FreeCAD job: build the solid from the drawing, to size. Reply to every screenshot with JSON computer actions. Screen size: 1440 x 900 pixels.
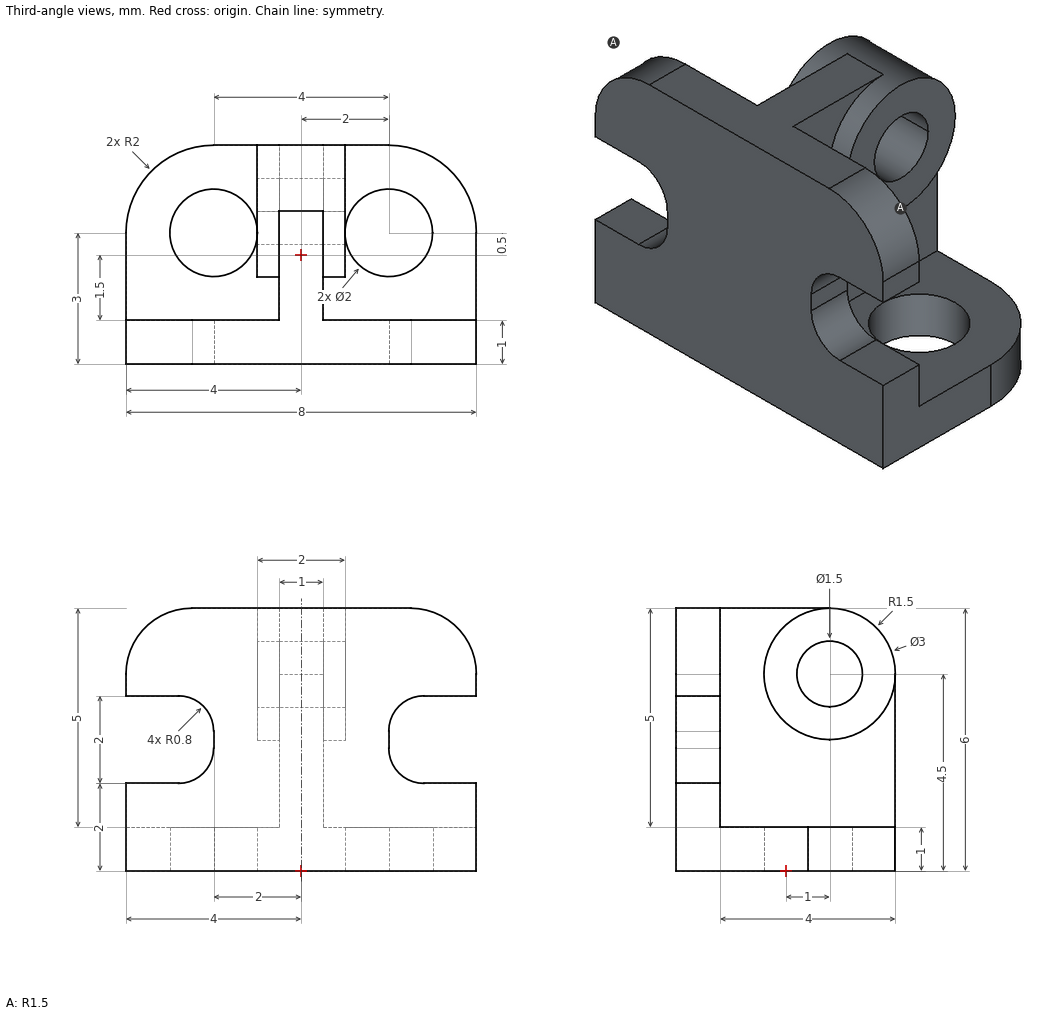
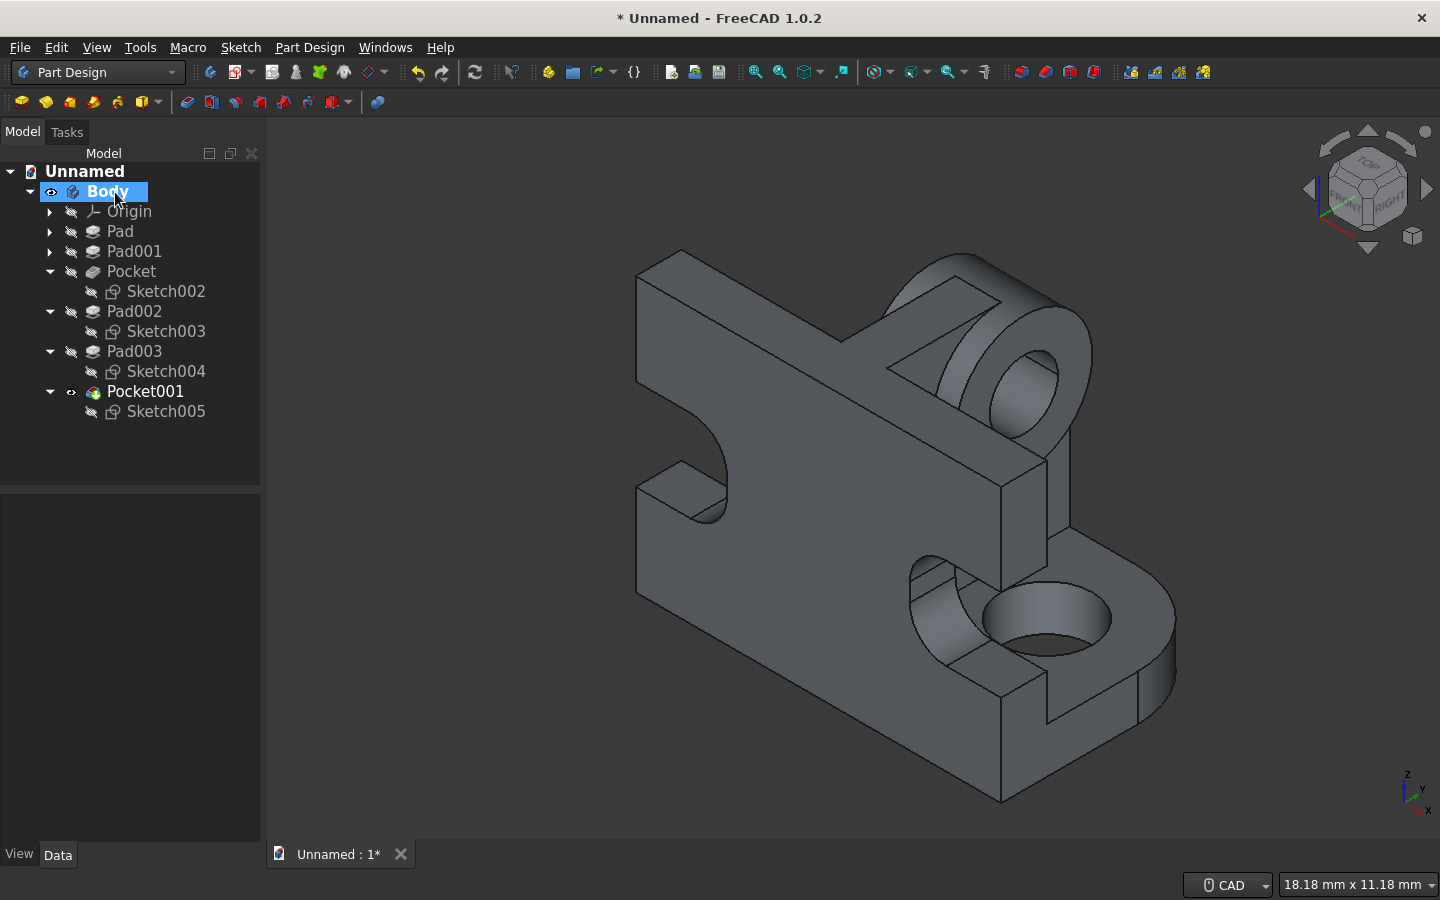
{"action": "left_click", "coordinate": [1024, 473]}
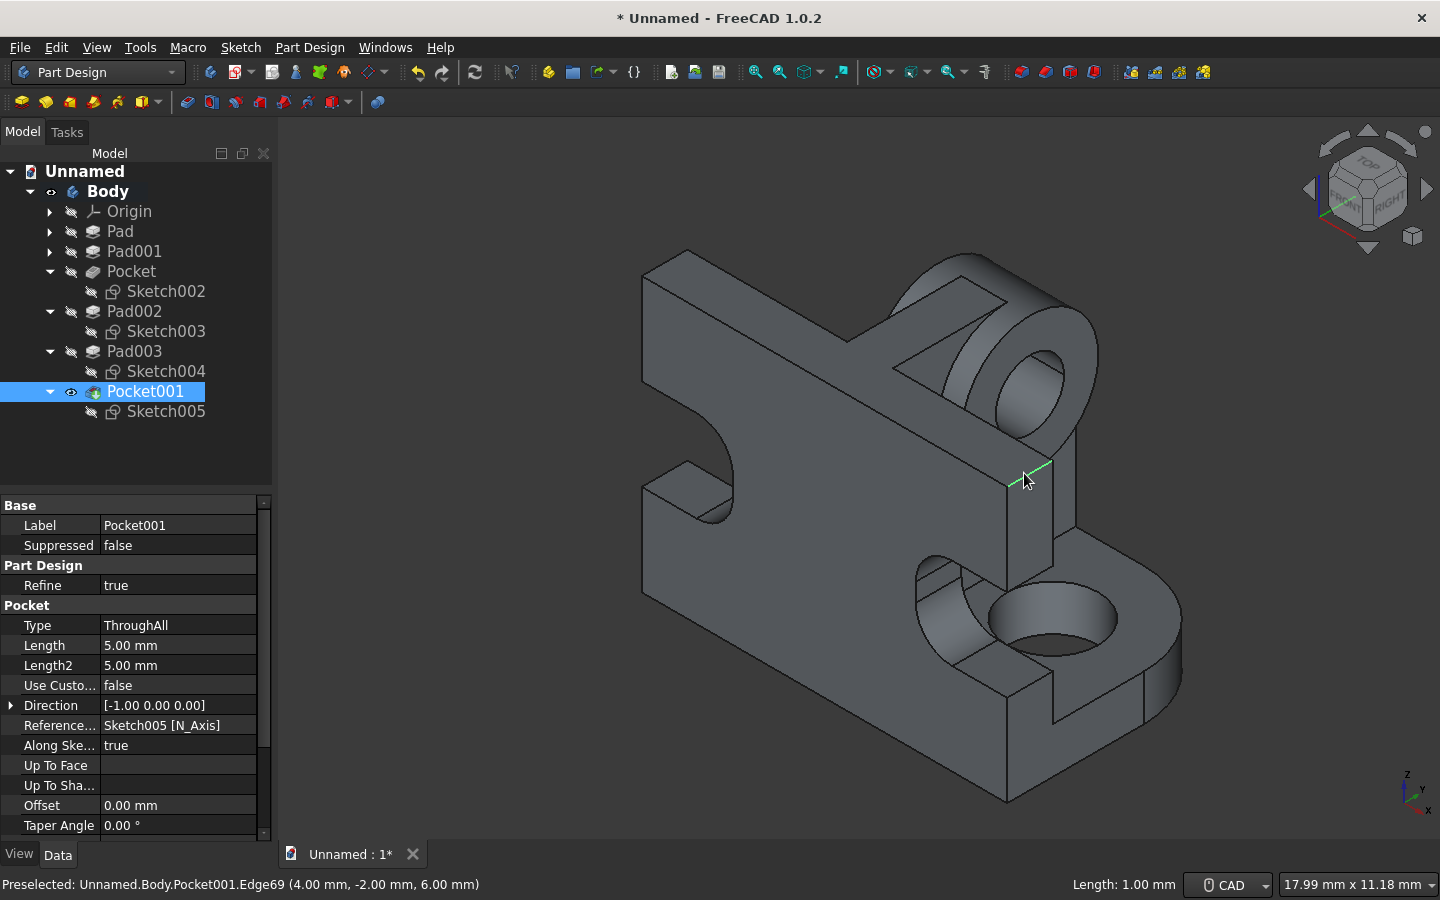
{"action": "key", "text": "2"}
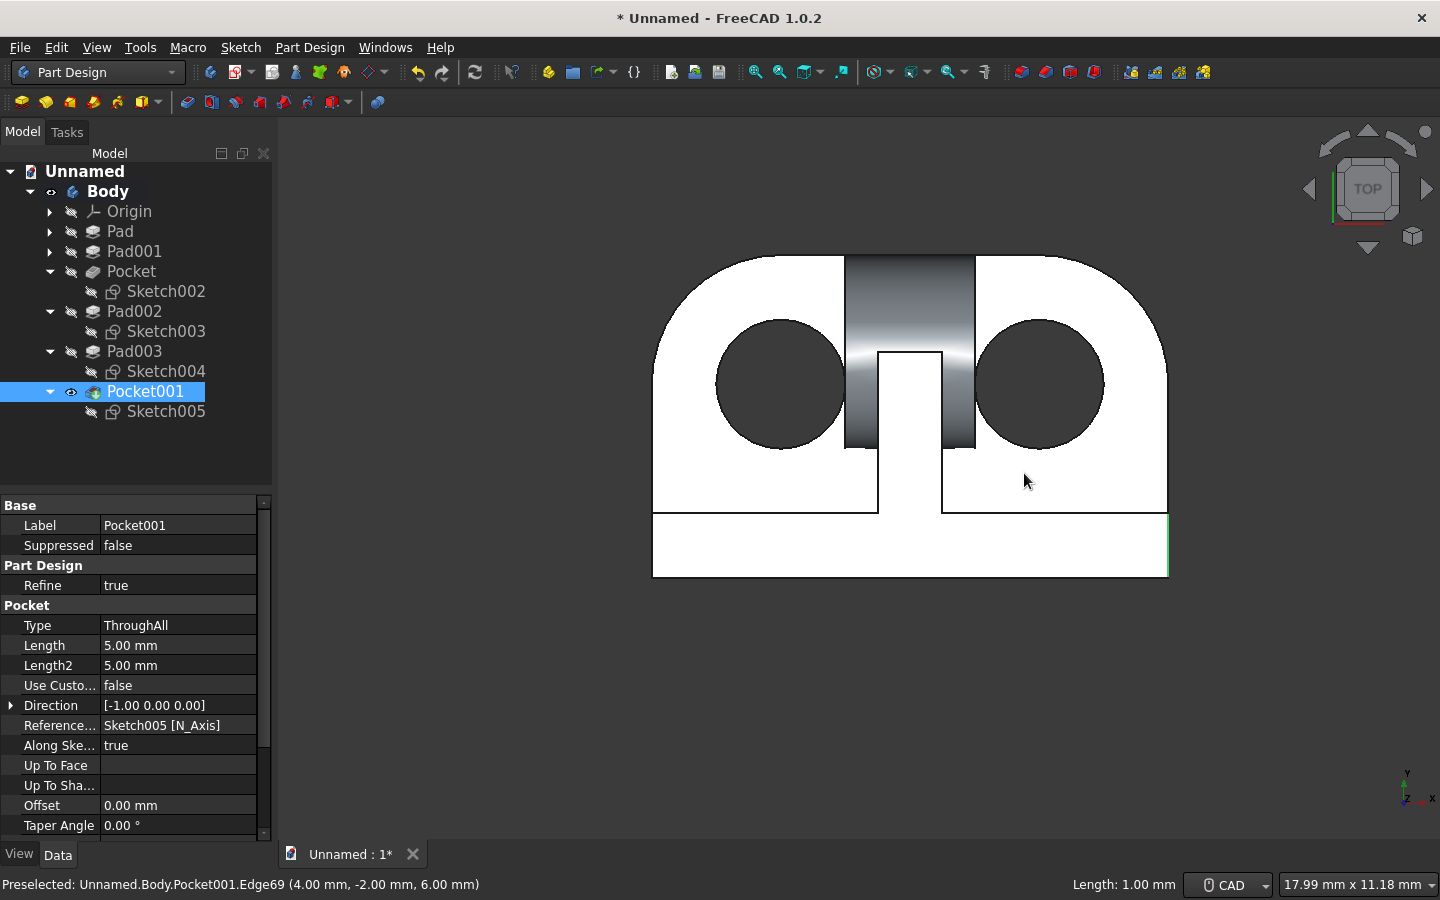
{"action": "left_click", "coordinate": [756, 72]}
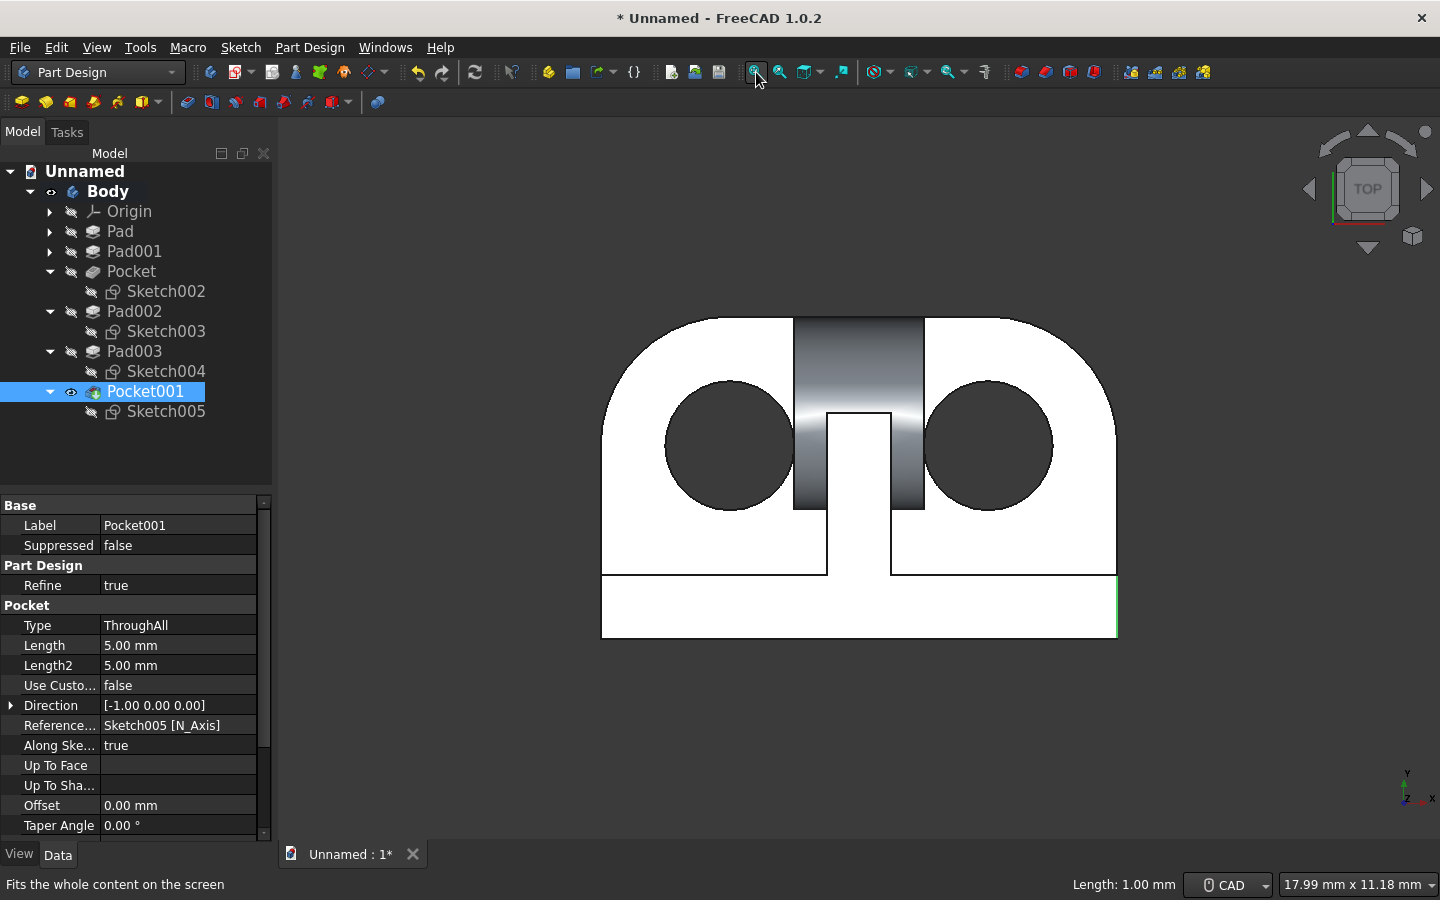
{"action": "left_click", "coordinate": [601, 606], "text": "ctrl"}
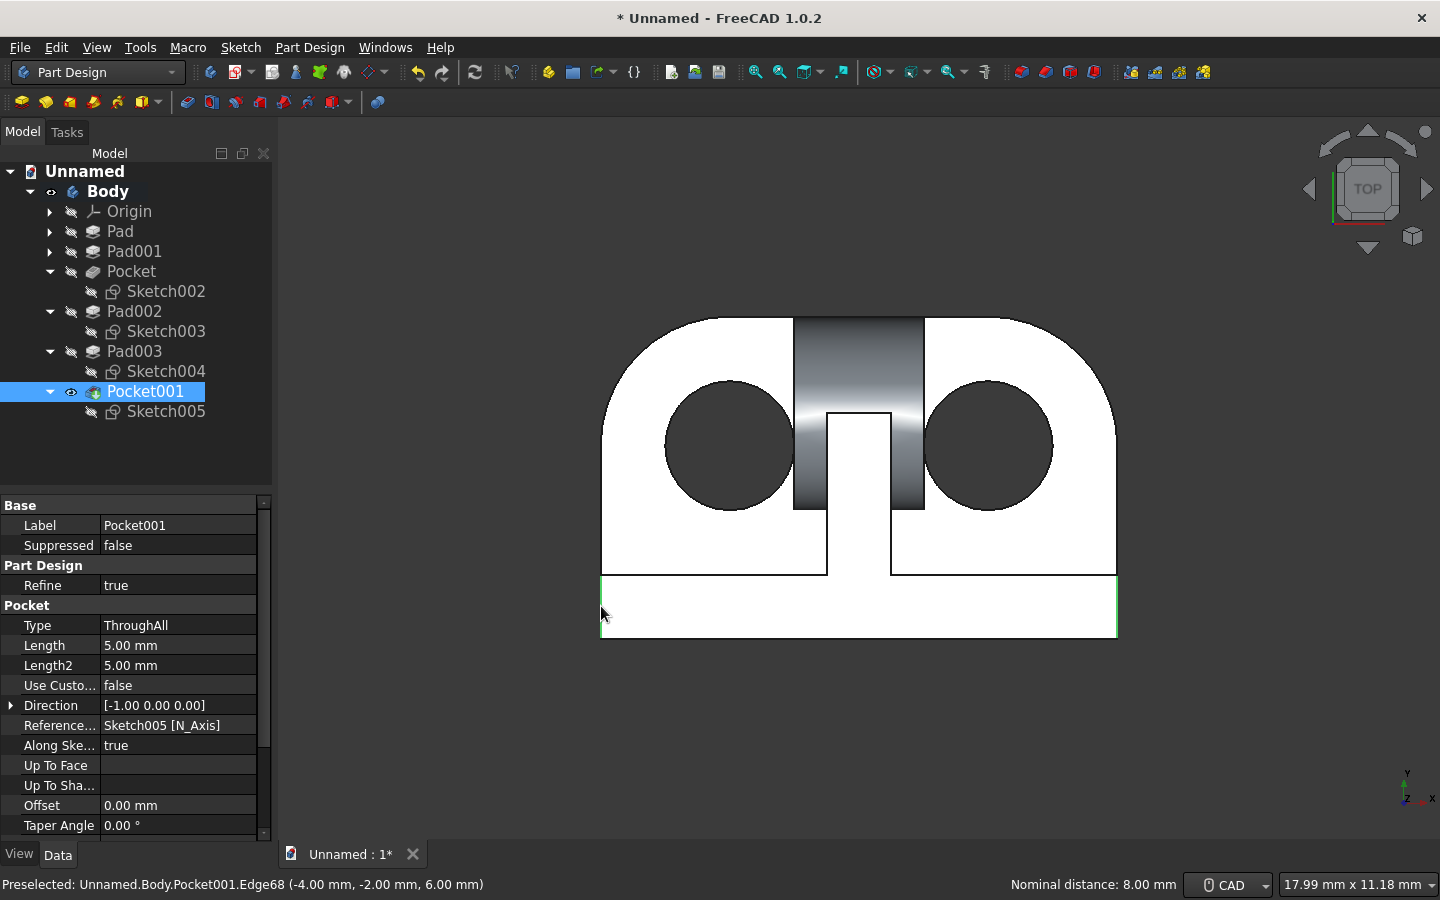
{"action": "left_click", "coordinate": [1022, 72]}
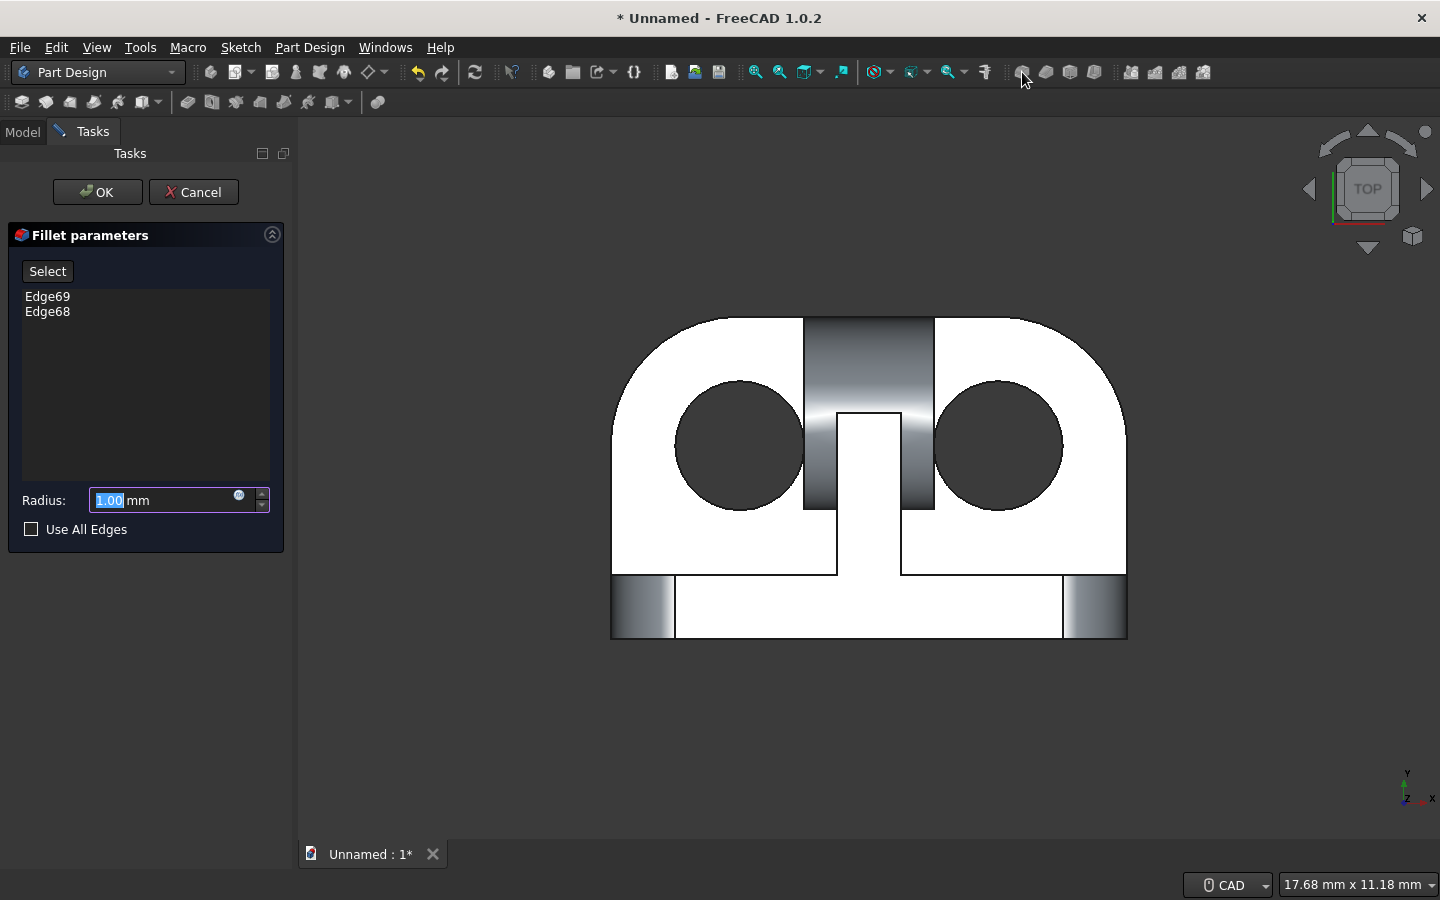
{"action": "type", "text": "1.5"}
{"action": "key", "text": "Tab"}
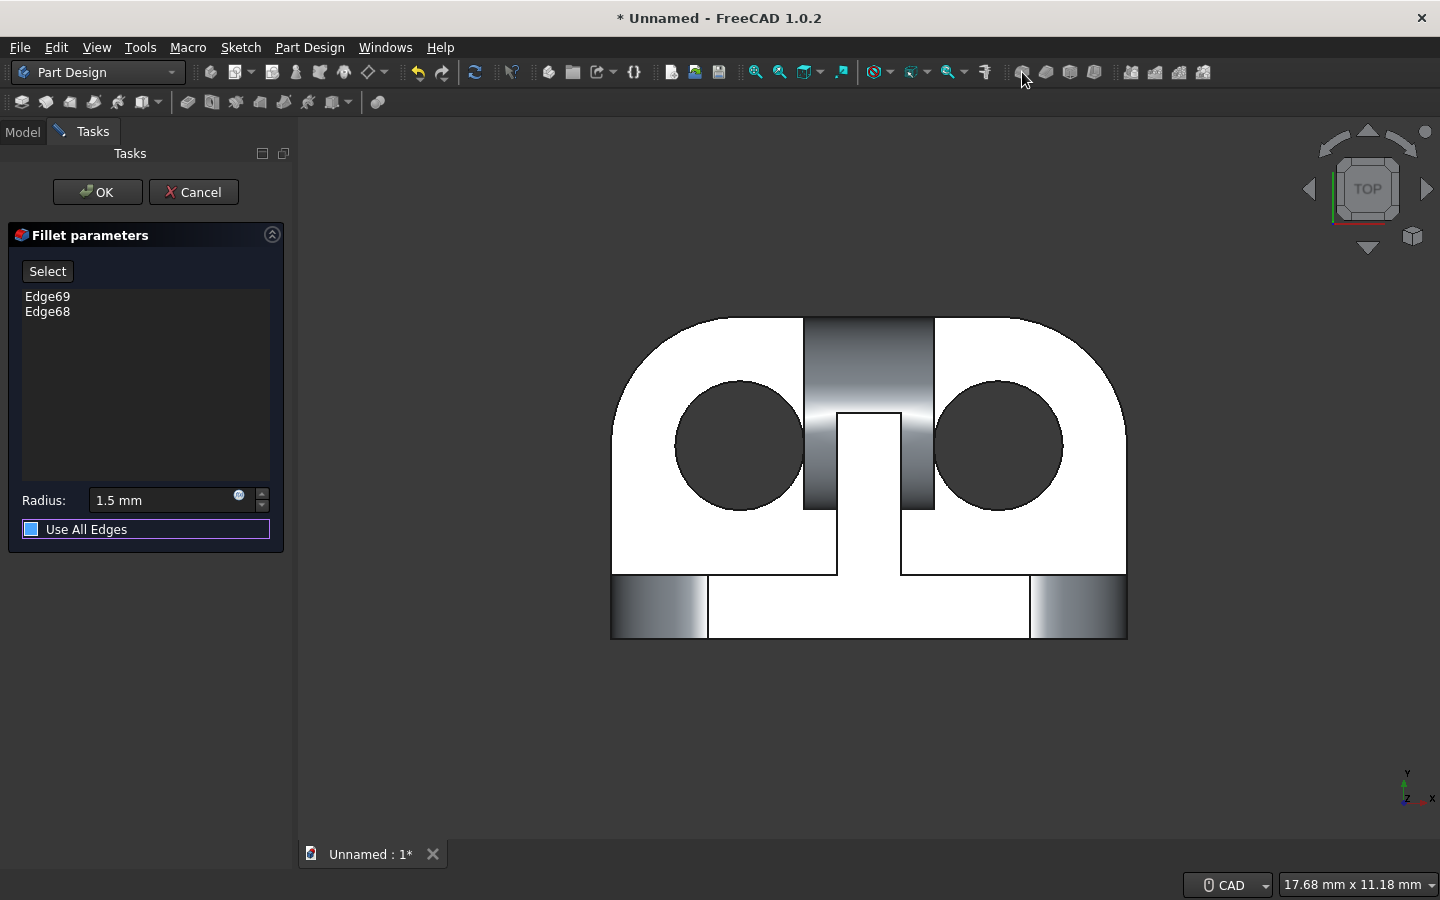
{"action": "left_click", "coordinate": [98, 192]}